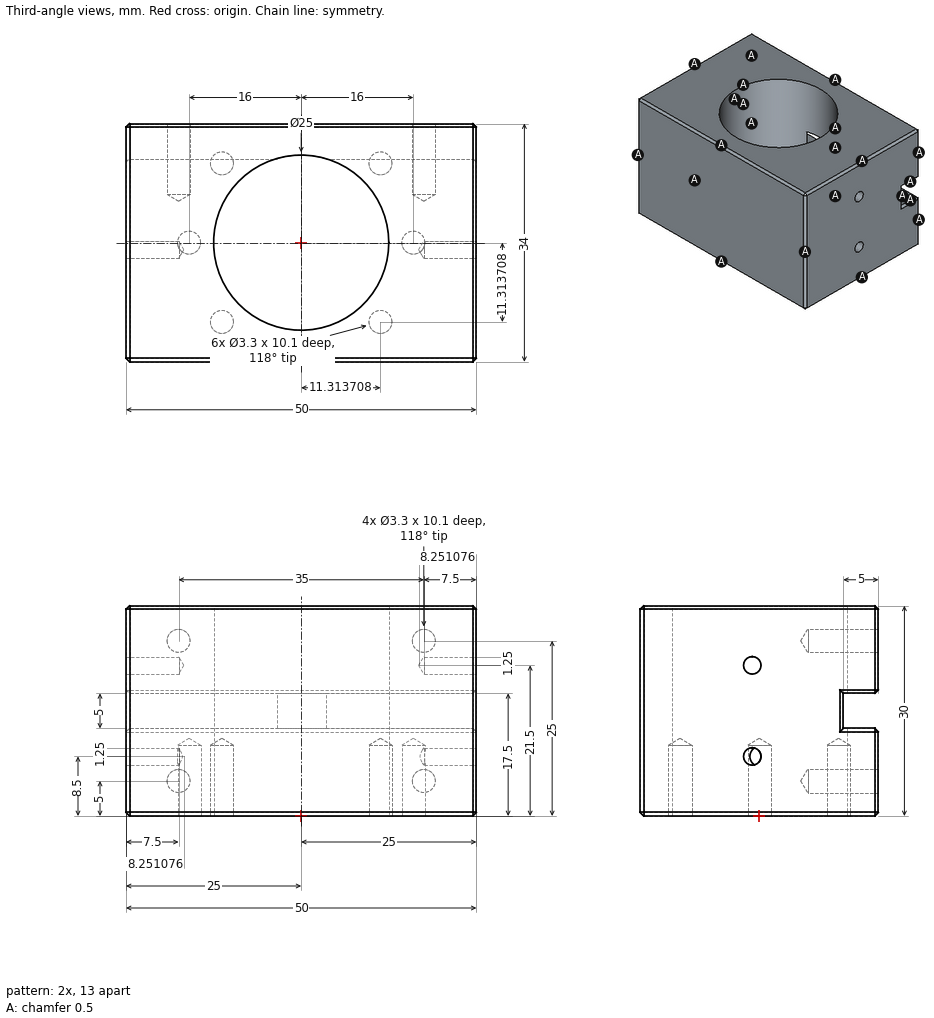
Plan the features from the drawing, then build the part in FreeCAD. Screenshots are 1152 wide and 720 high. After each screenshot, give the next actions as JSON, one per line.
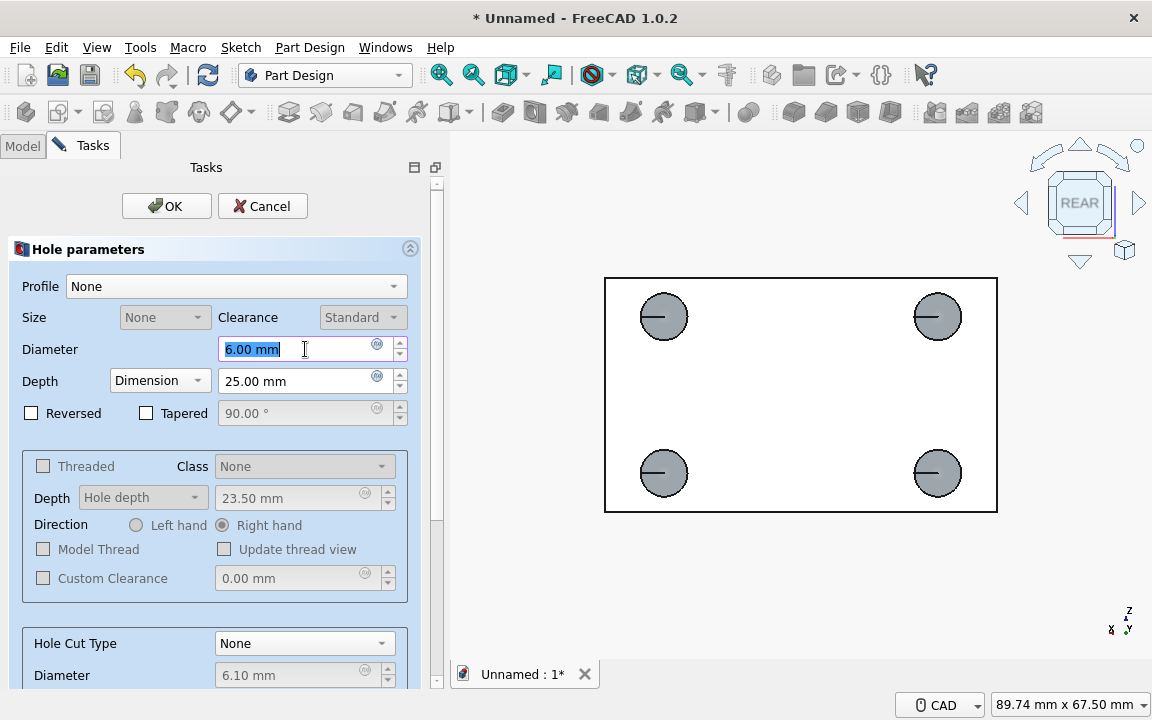
{"action": "type", "text": "3.3"}
{"action": "key", "text": "Tab"}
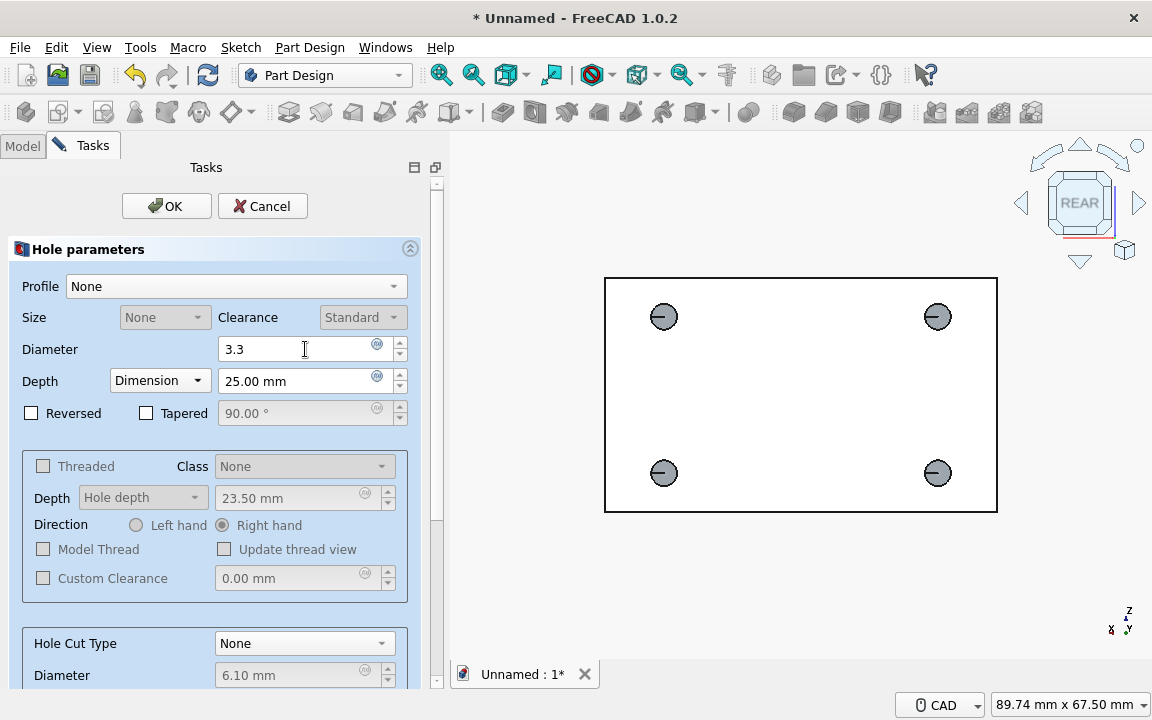
{"action": "triple_click", "coordinate": [305, 381]}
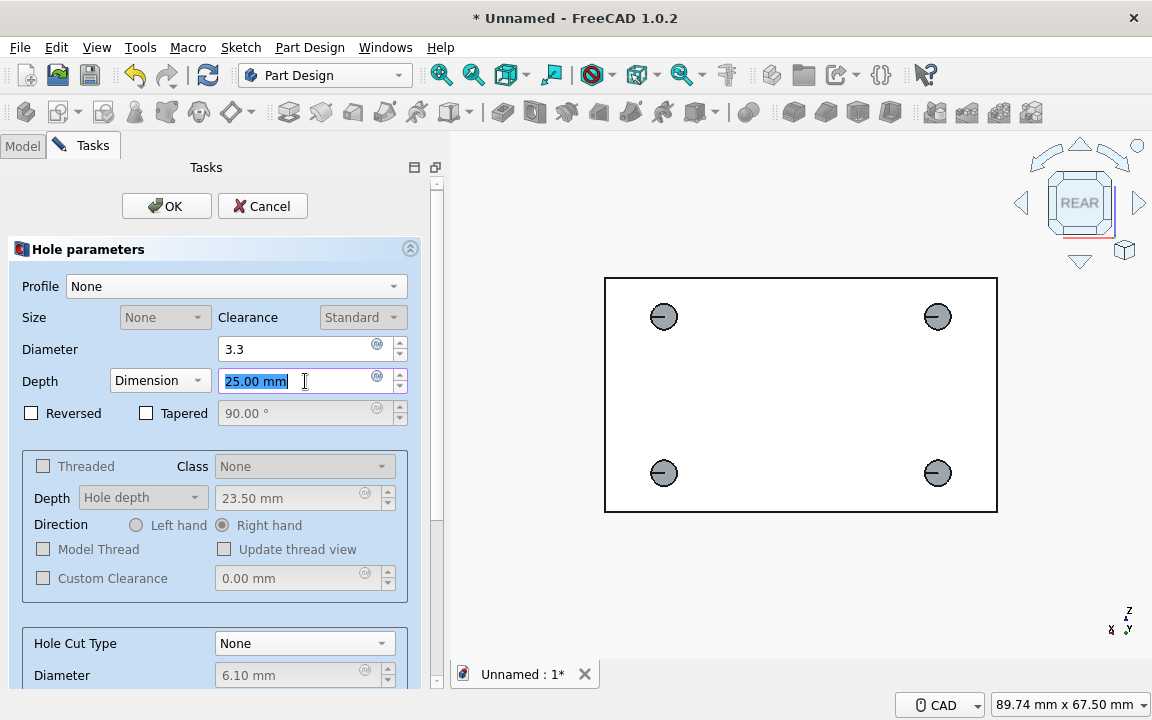
{"action": "type", "text": "10.1"}
{"action": "key", "text": "Tab"}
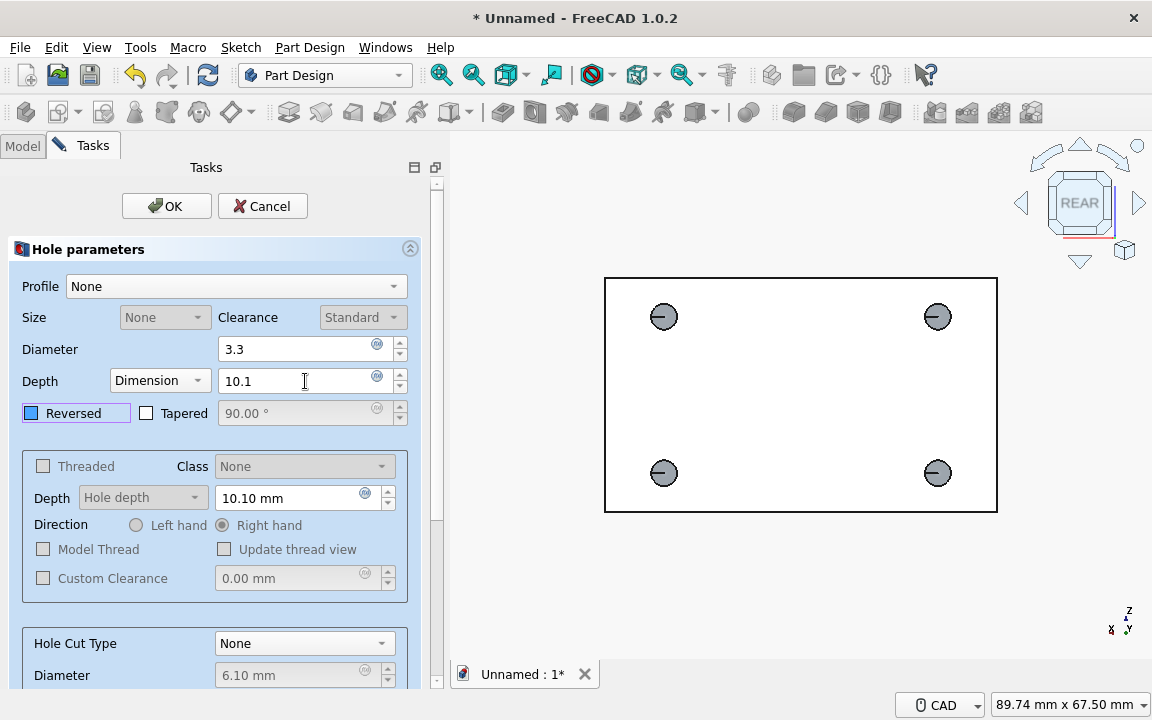
{"action": "left_click", "coordinate": [167, 206]}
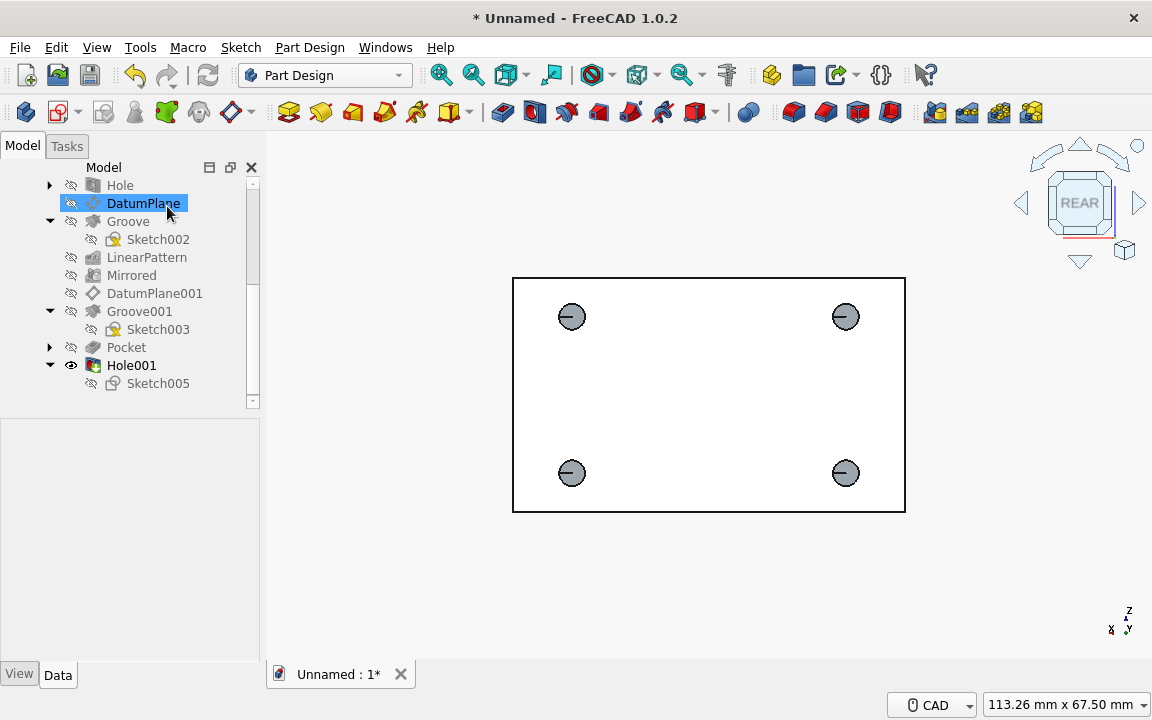
{"action": "key", "text": "v f"}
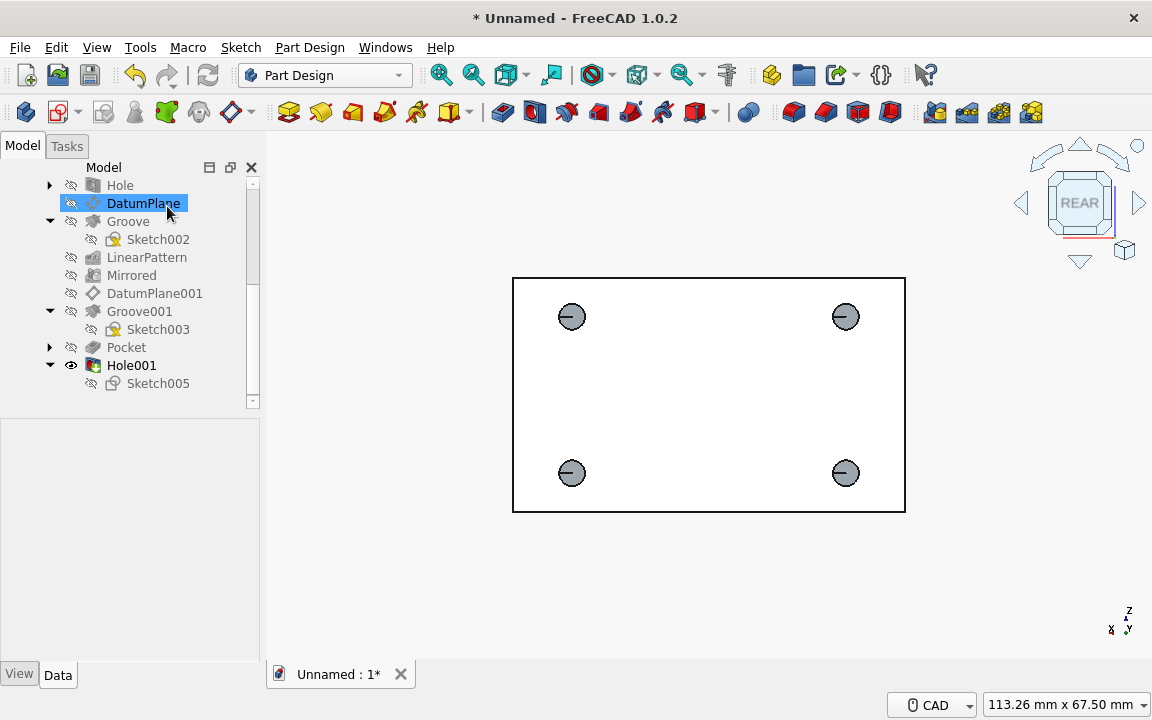
{"action": "left_click", "coordinate": [709, 394]}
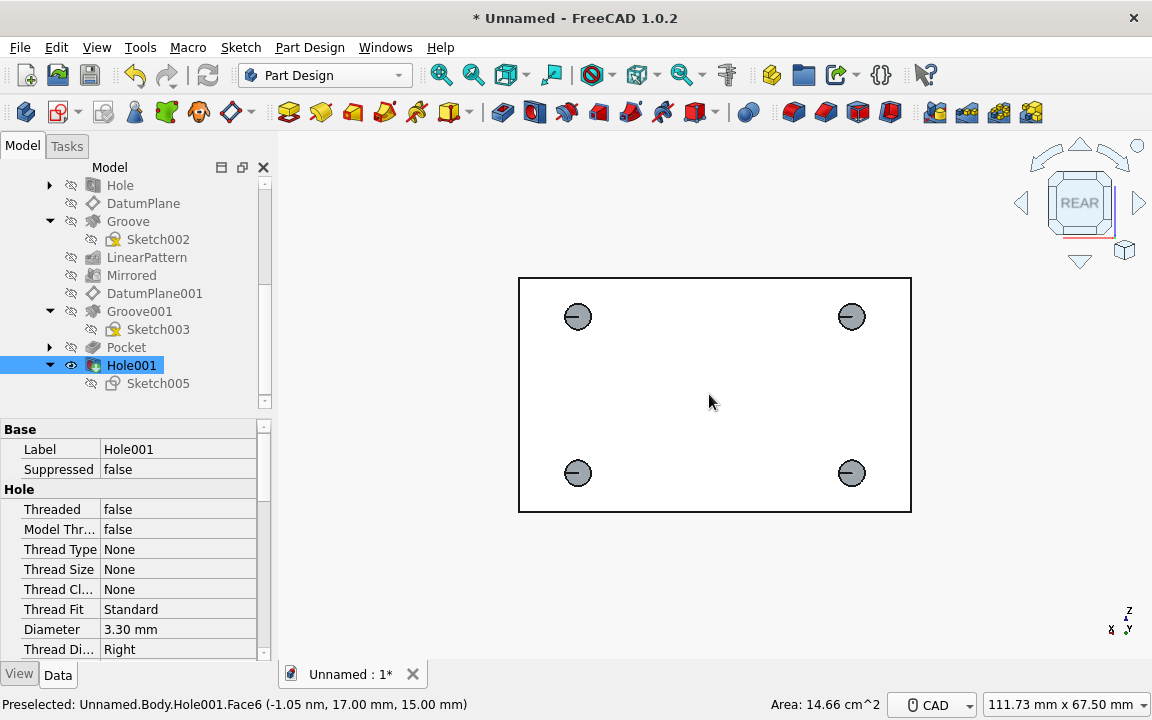
{"action": "left_click", "coordinate": [58, 112]}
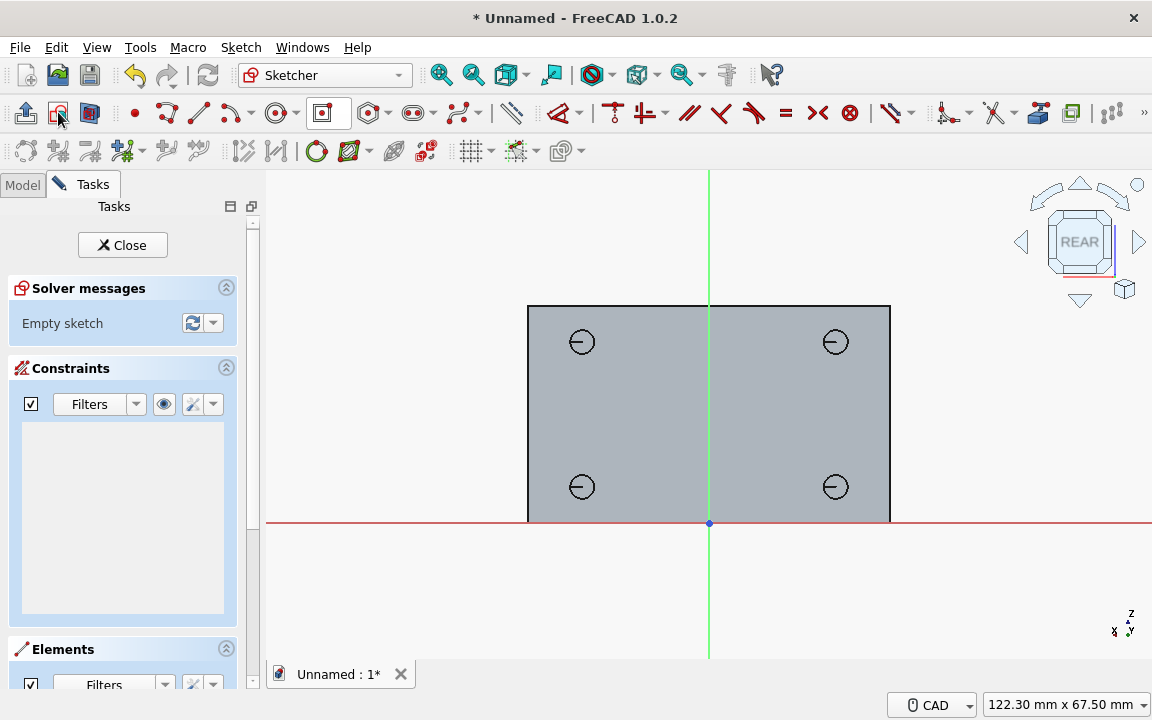
{"action": "scroll", "coordinate": [848, 552], "scroll_direction": "up", "scroll_amount": 2}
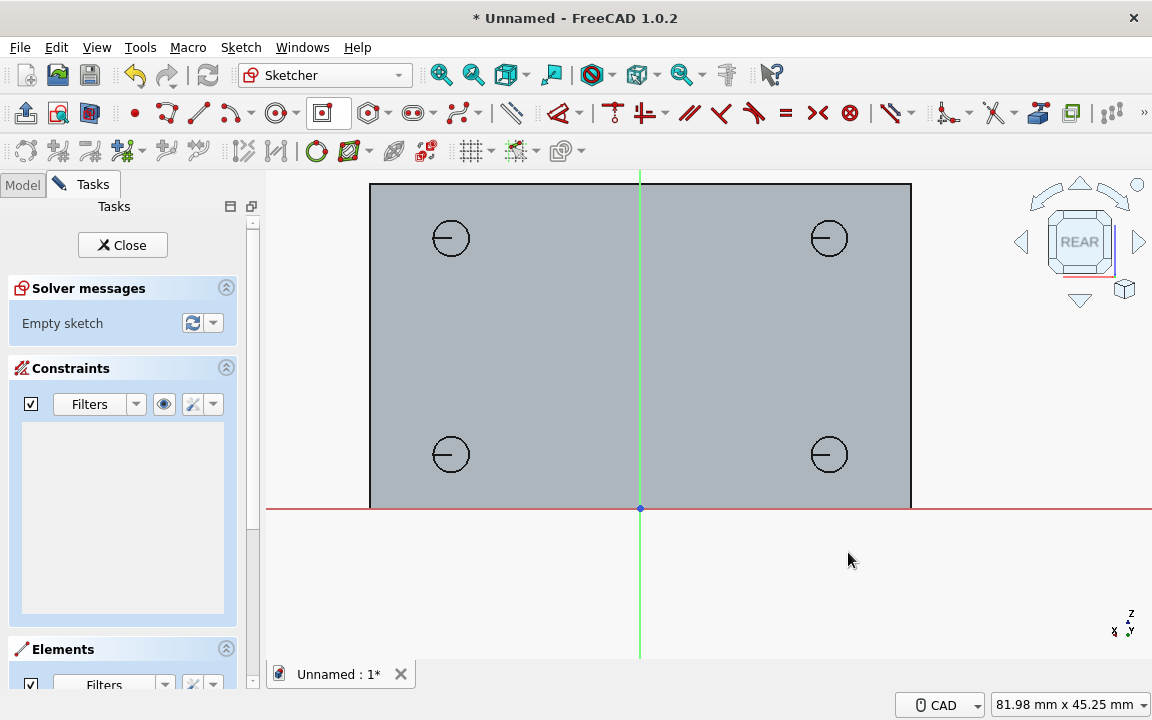
{"action": "key", "text": "g r"}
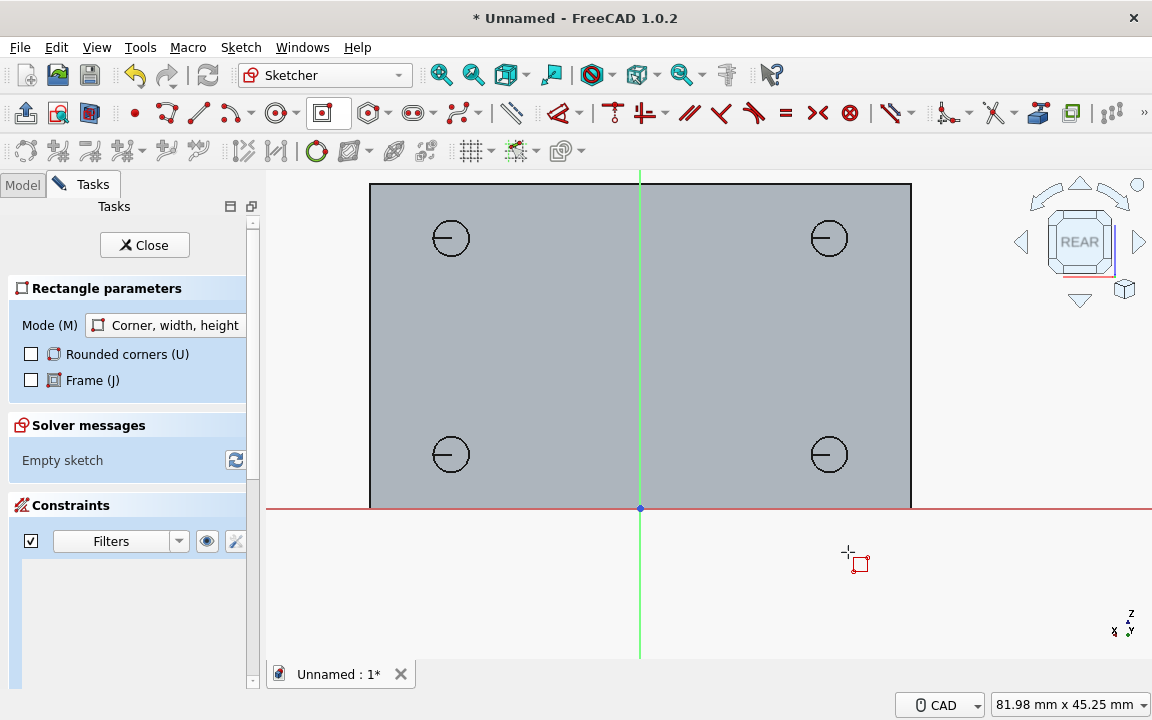
{"action": "left_click", "coordinate": [370, 319]}
{"action": "mouse_move", "coordinate": [911, 374]}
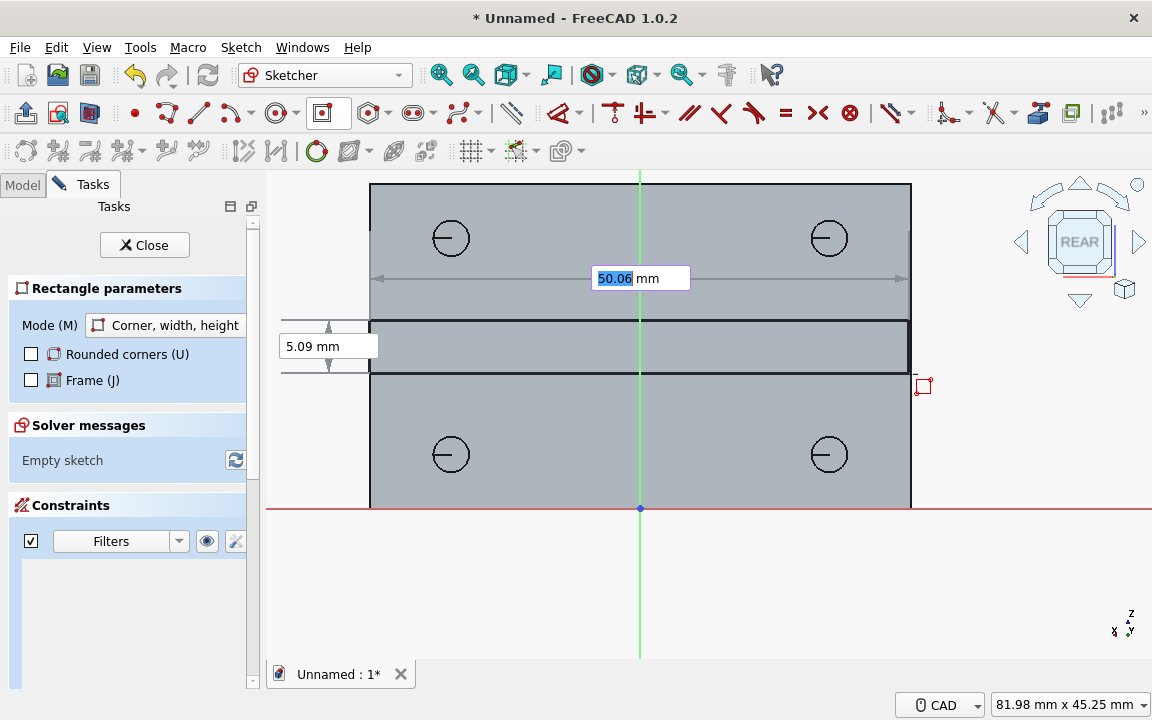
{"action": "type", "text": "50"}
{"action": "key", "text": "Tab"}
{"action": "type", "text": "5"}
{"action": "key", "text": "Return"}
{"action": "key", "text": "Escape"}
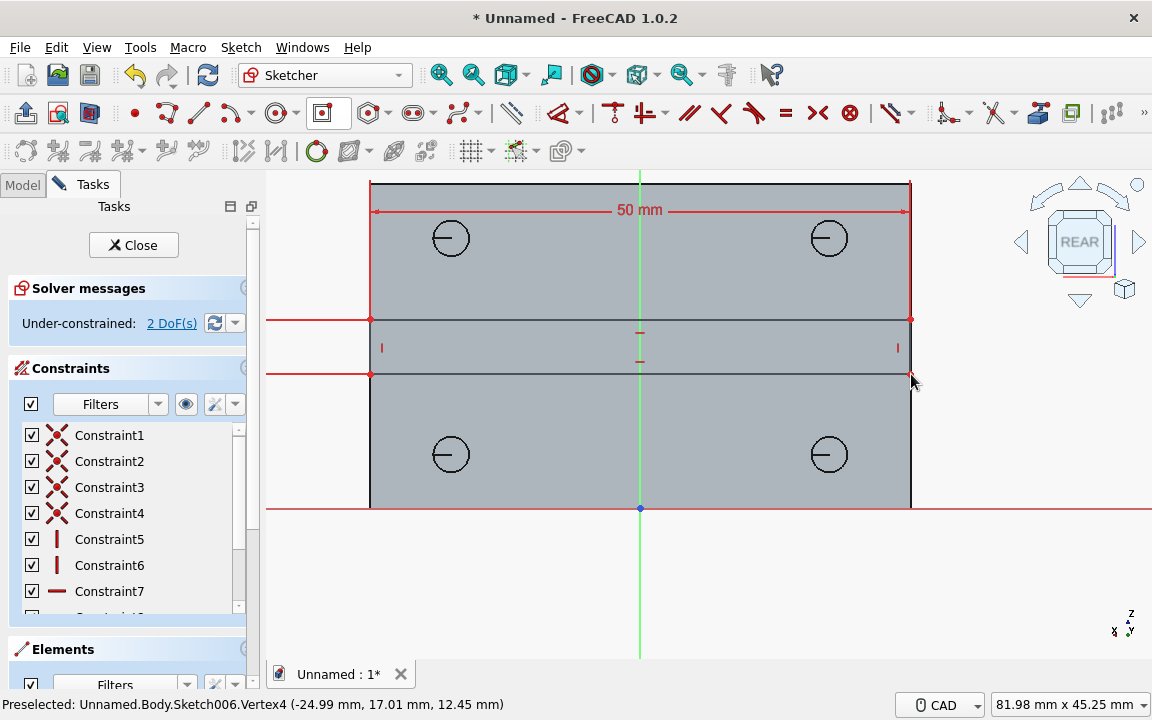
{"action": "left_click", "coordinate": [558, 114]}